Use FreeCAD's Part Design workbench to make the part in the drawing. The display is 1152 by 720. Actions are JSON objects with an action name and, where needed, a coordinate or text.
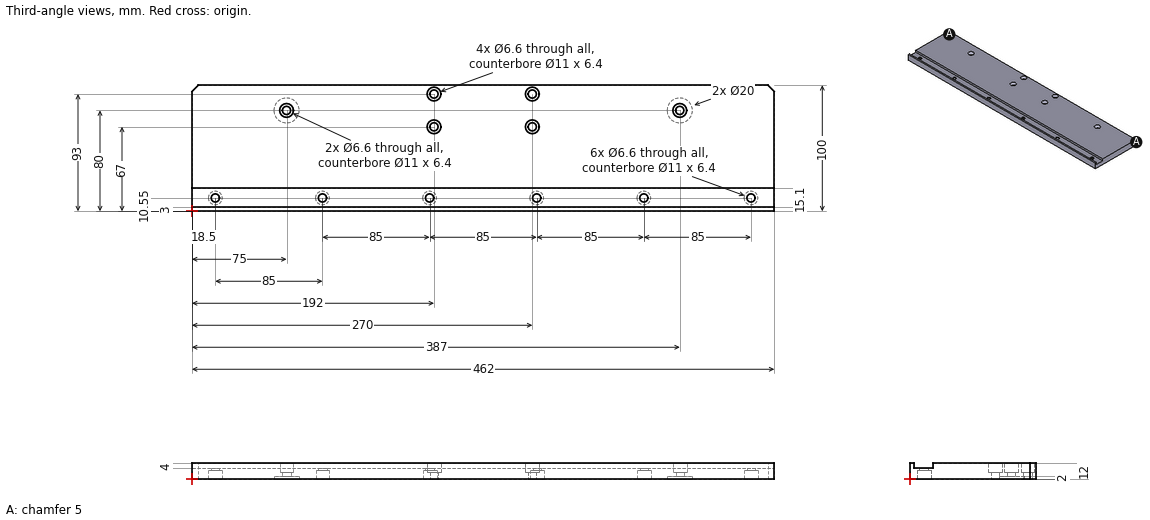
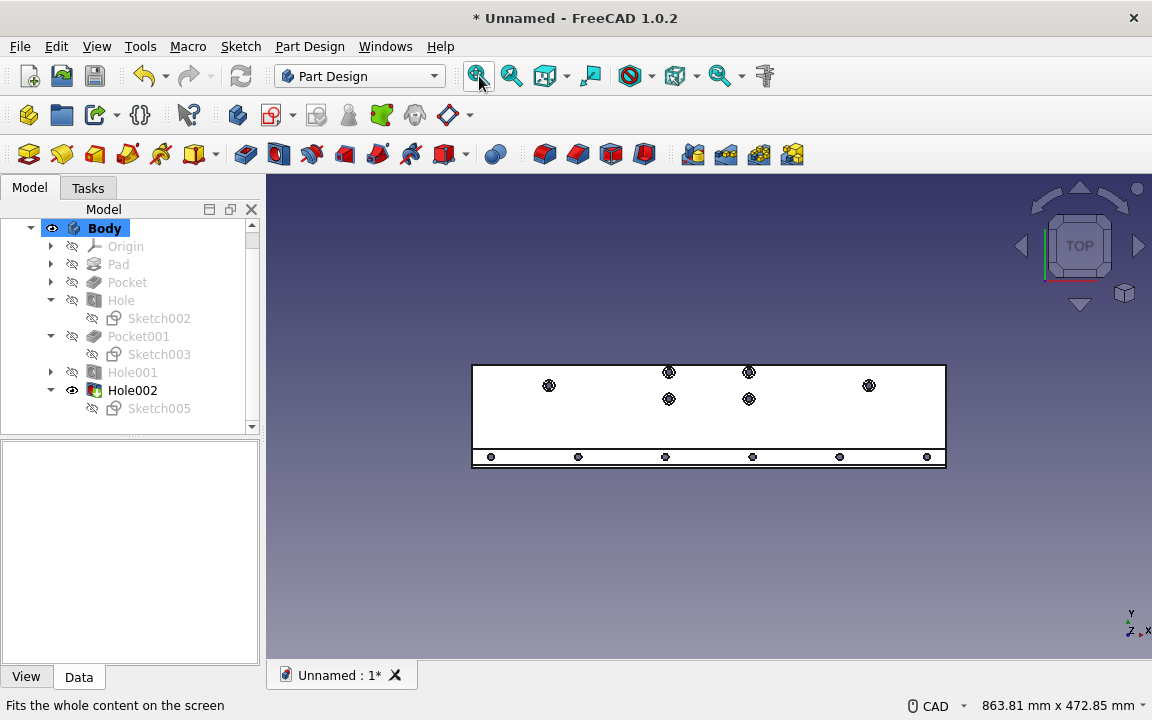
{"action": "scroll", "coordinate": [472, 364], "scroll_direction": "up", "scroll_amount": 6}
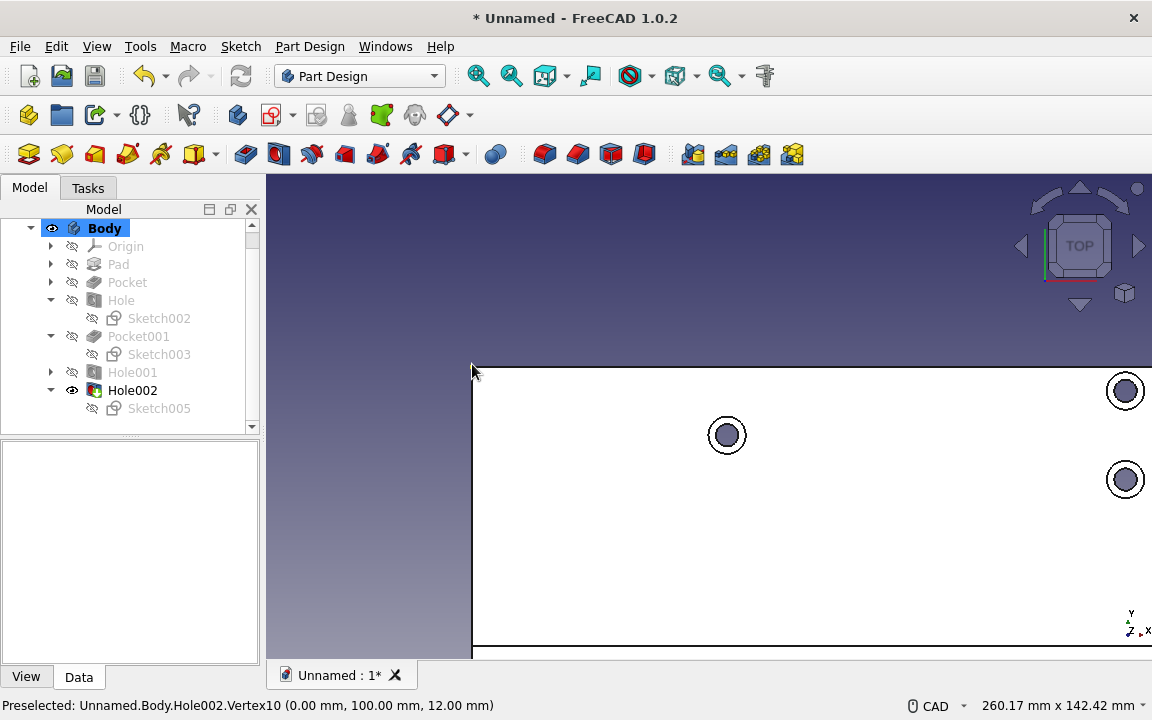
{"action": "left_click", "coordinate": [479, 76]}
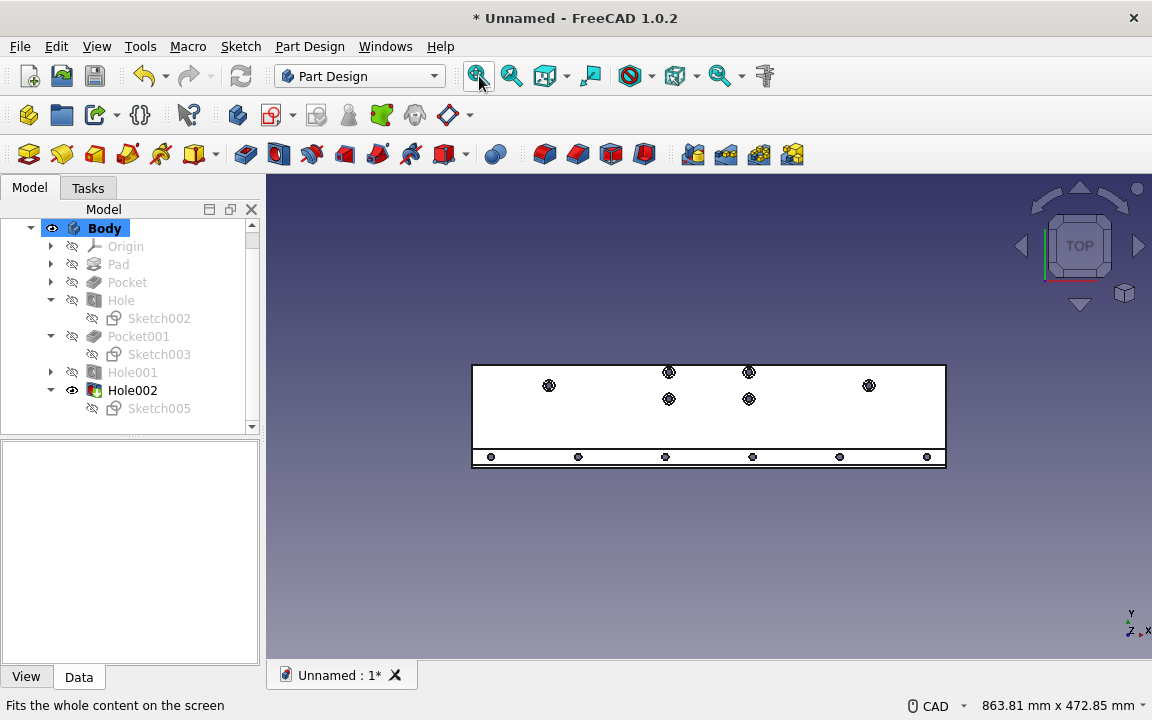
{"action": "key", "text": "1"}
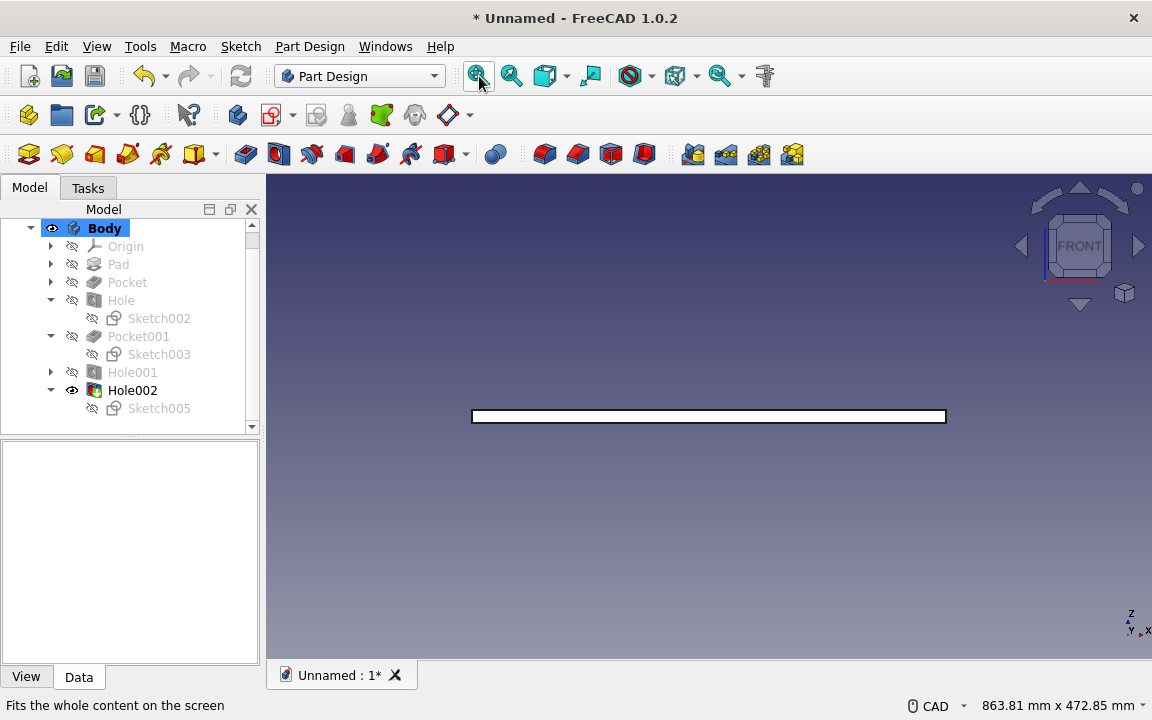
{"action": "scroll", "coordinate": [472, 416], "scroll_direction": "up", "scroll_amount": 6}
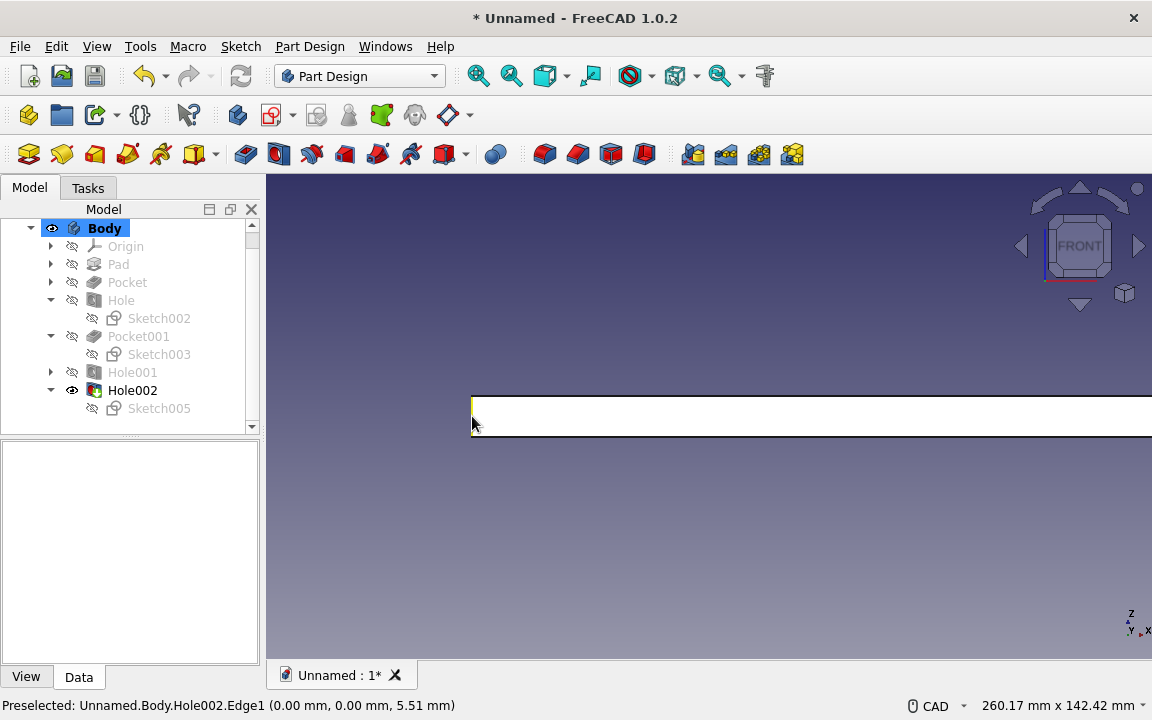
{"action": "left_click", "coordinate": [479, 76]}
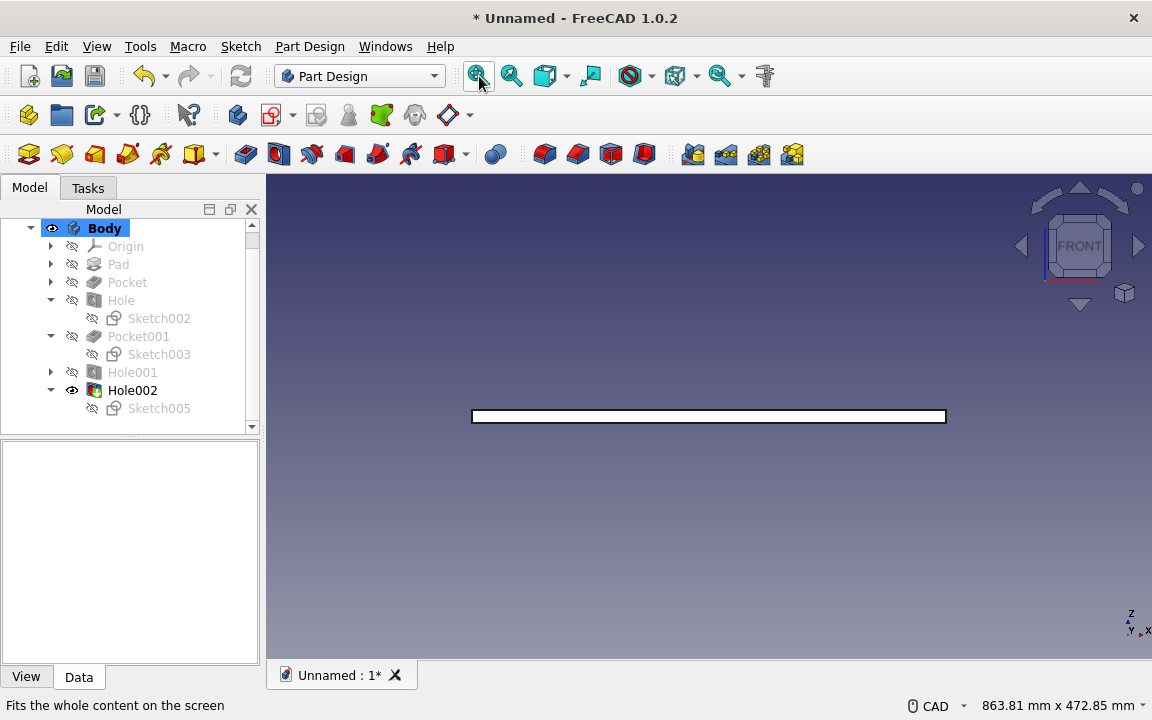
{"action": "key", "text": "3"}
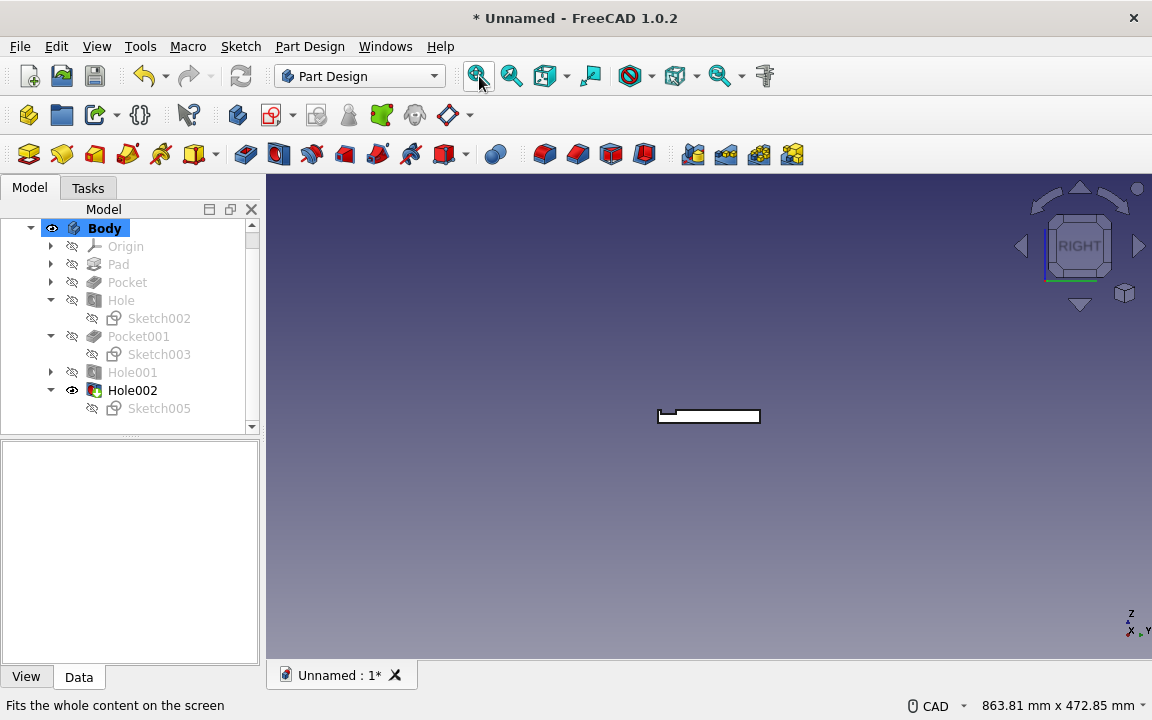
{"action": "left_click", "coordinate": [479, 76]}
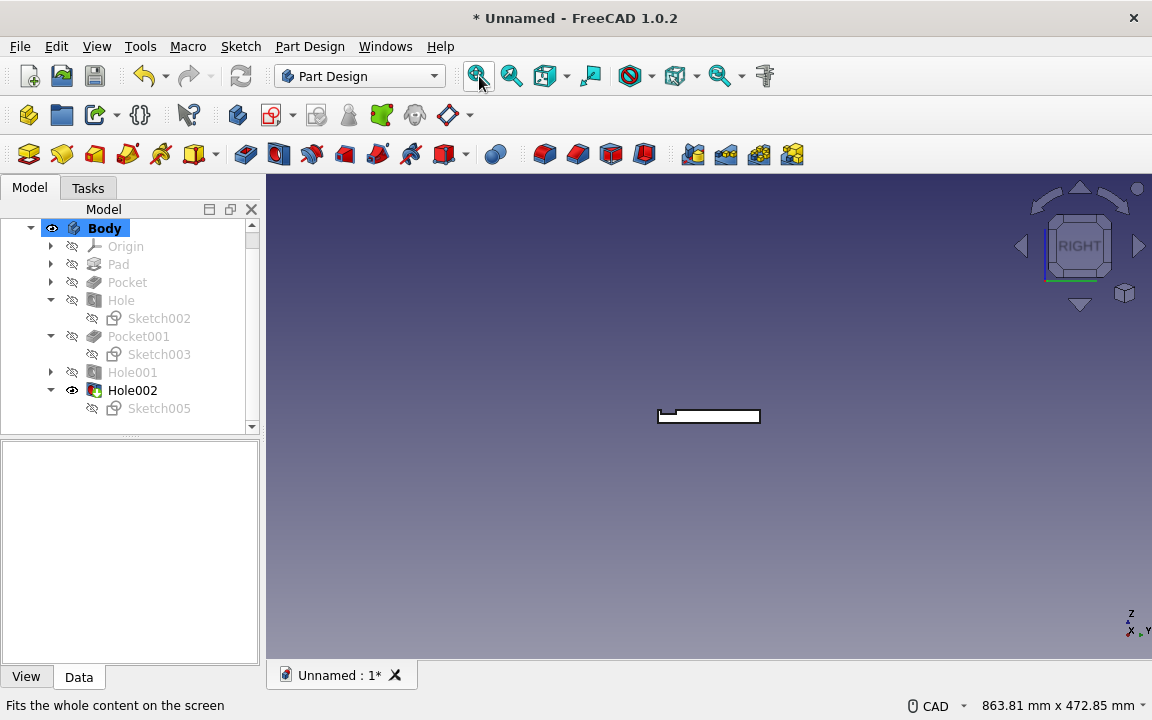
{"action": "scroll", "coordinate": [760, 415], "scroll_direction": "up", "scroll_amount": 6}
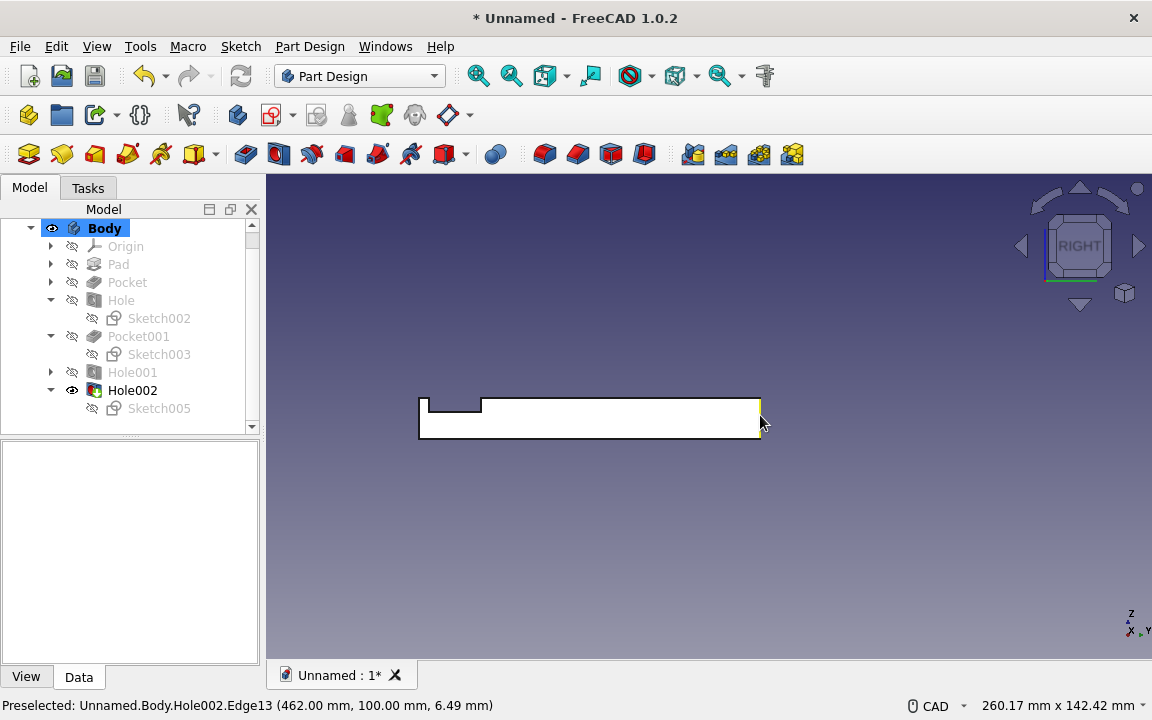
{"action": "left_click", "coordinate": [760, 418]}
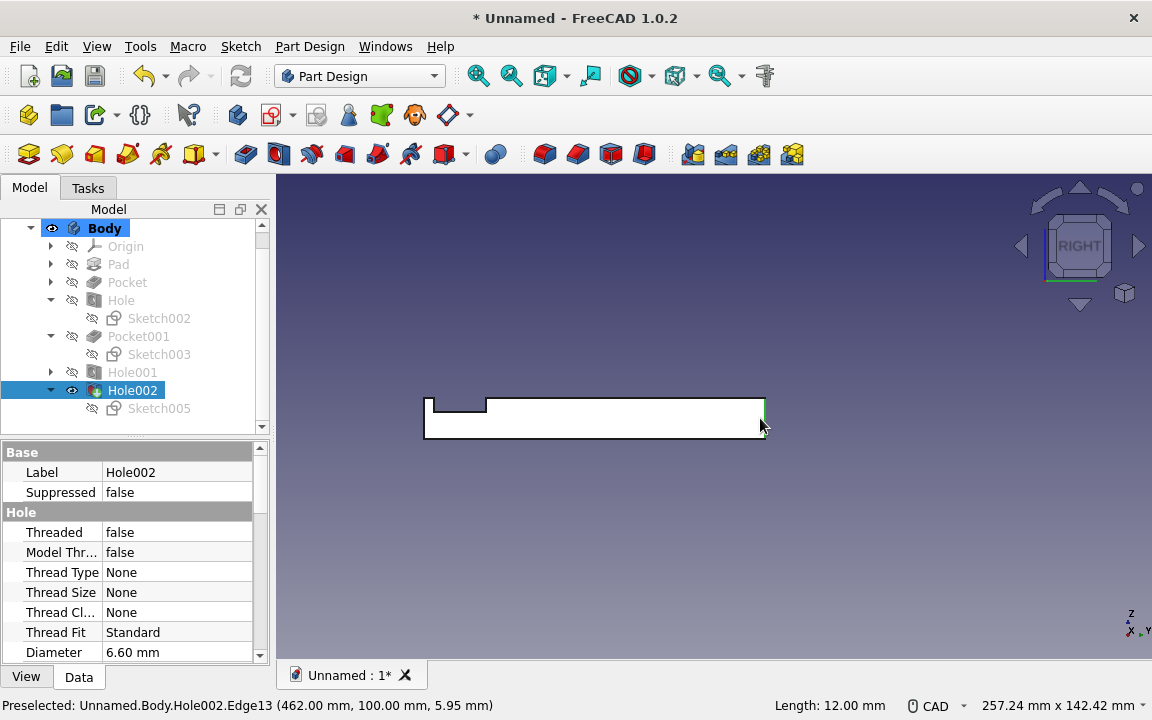
{"action": "left_click", "coordinate": [479, 76]}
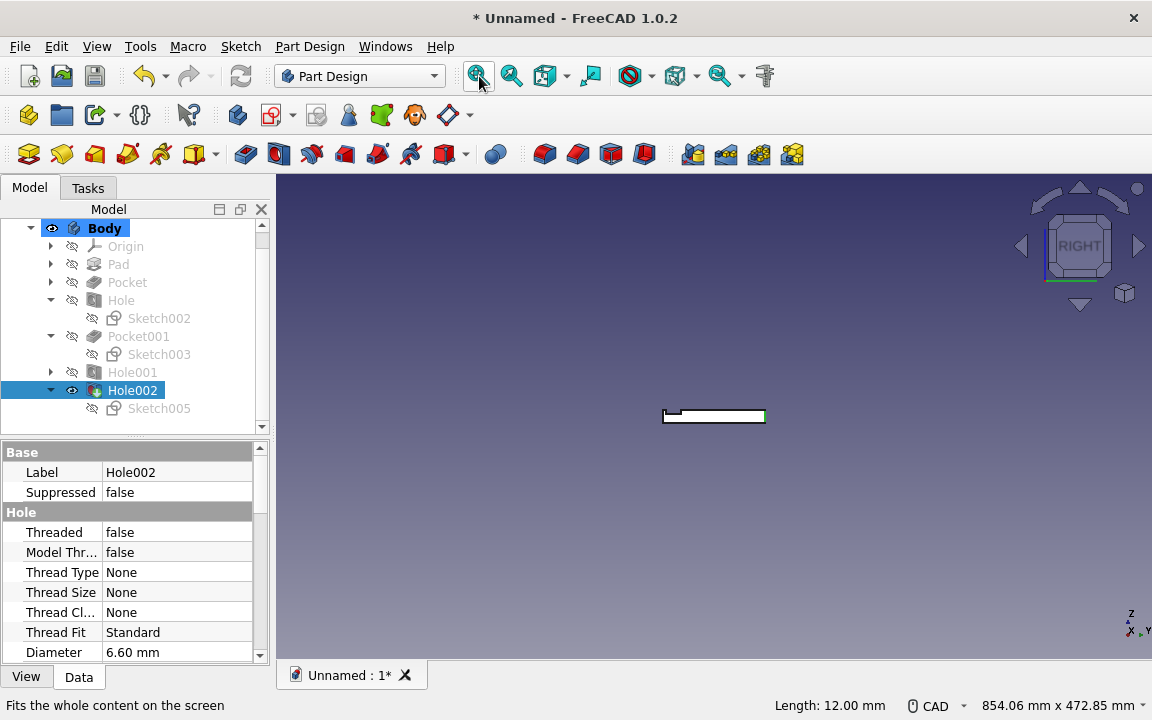
{"action": "key", "text": "5"}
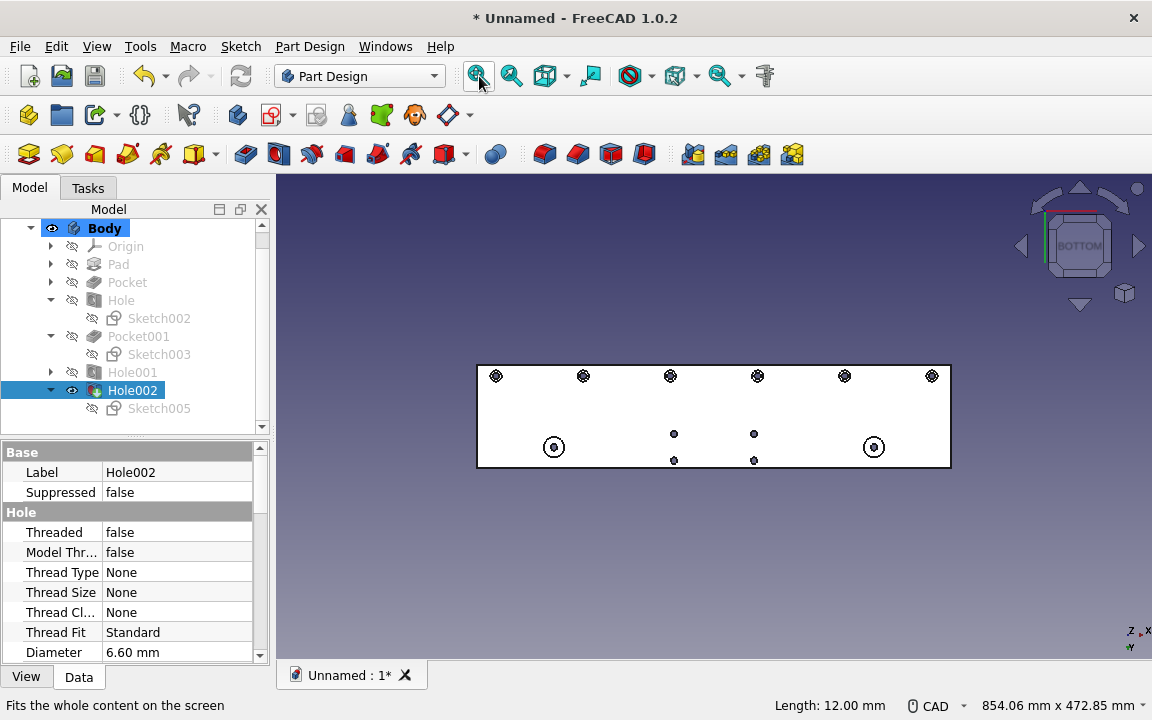
{"action": "scroll", "coordinate": [477, 467], "scroll_direction": "up", "scroll_amount": 6}